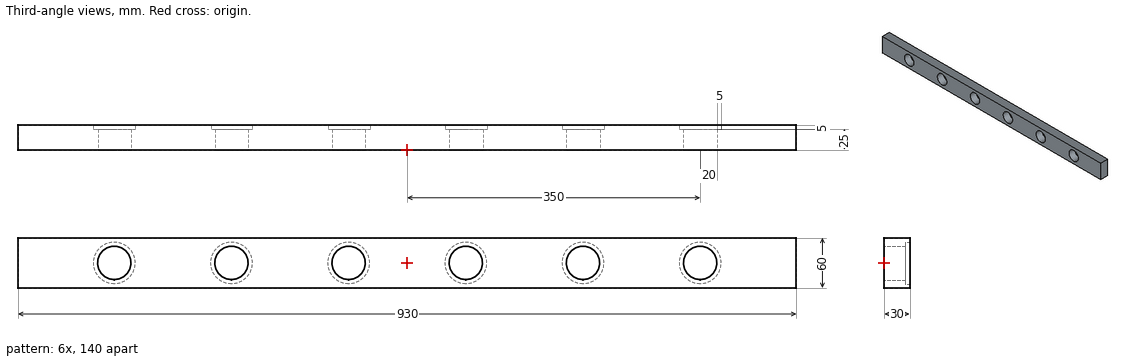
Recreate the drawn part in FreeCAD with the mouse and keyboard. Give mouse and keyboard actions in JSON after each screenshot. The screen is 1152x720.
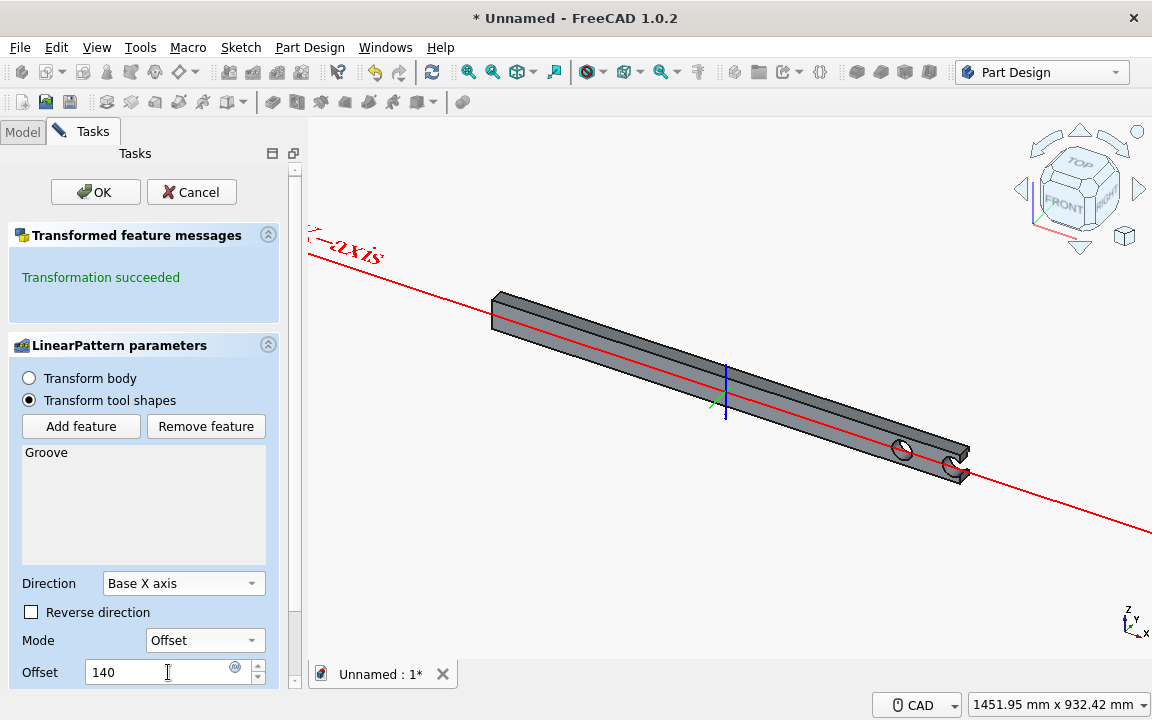
{"action": "scroll", "coordinate": [295, 426], "scroll_direction": "down", "scroll_amount": 2}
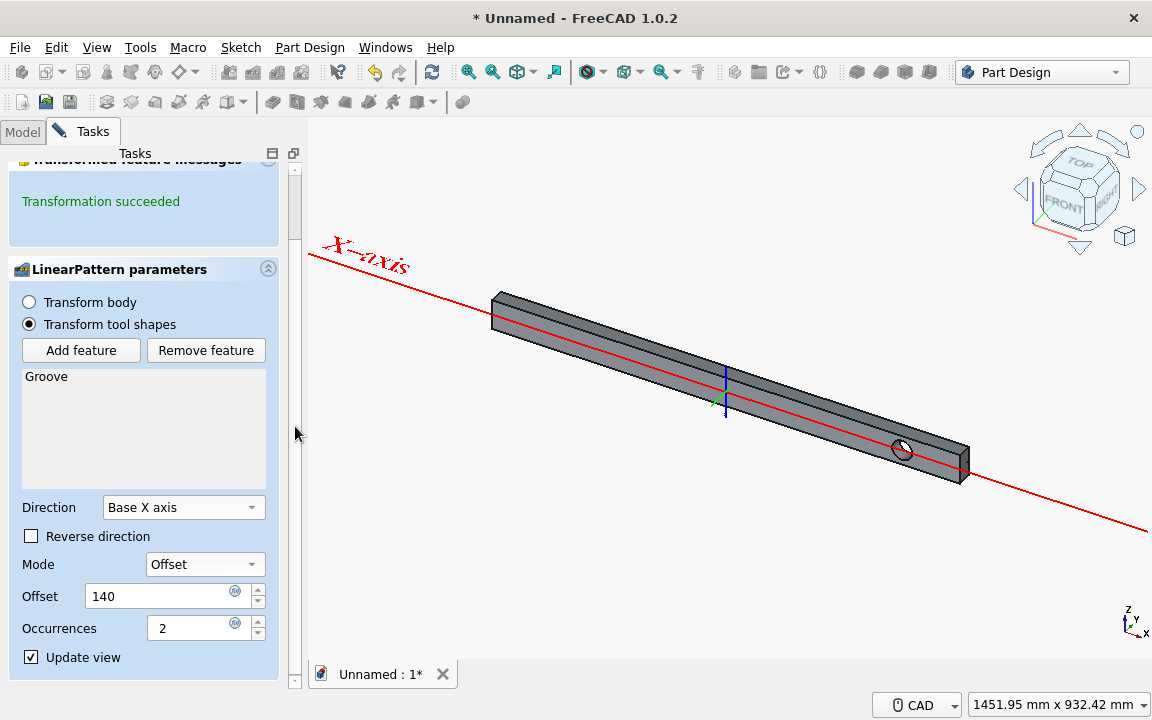
{"action": "triple_click", "coordinate": [198, 628]}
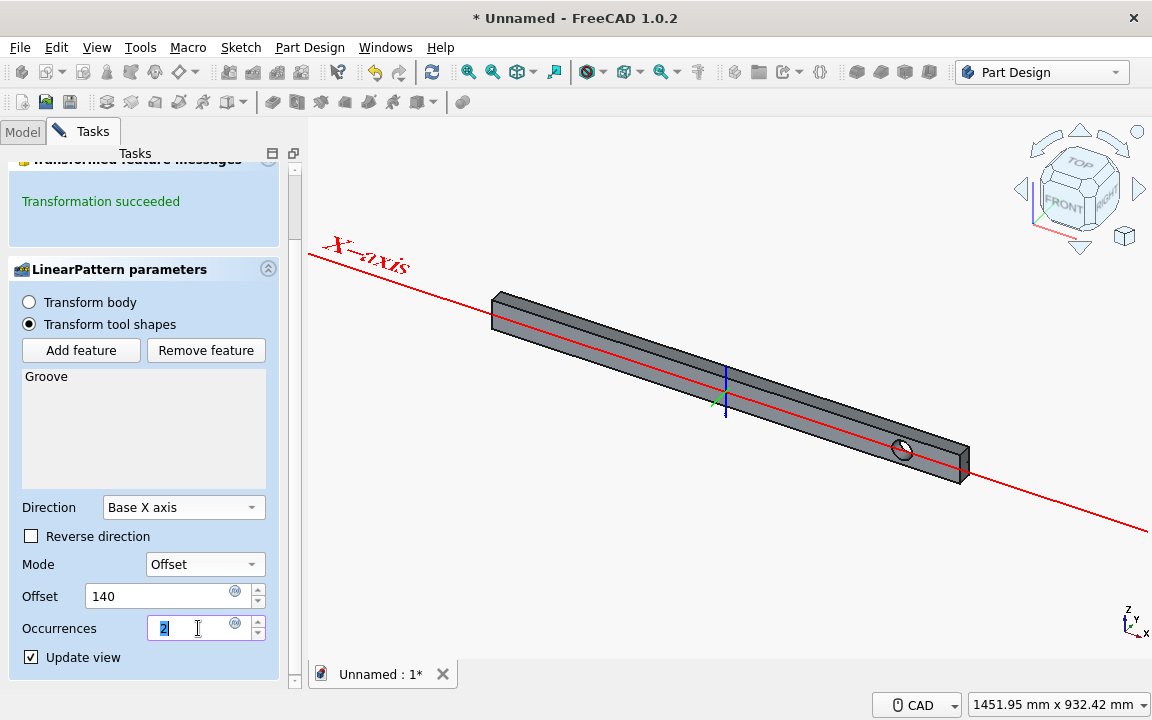
{"action": "type", "text": "6"}
{"action": "key", "text": "Tab"}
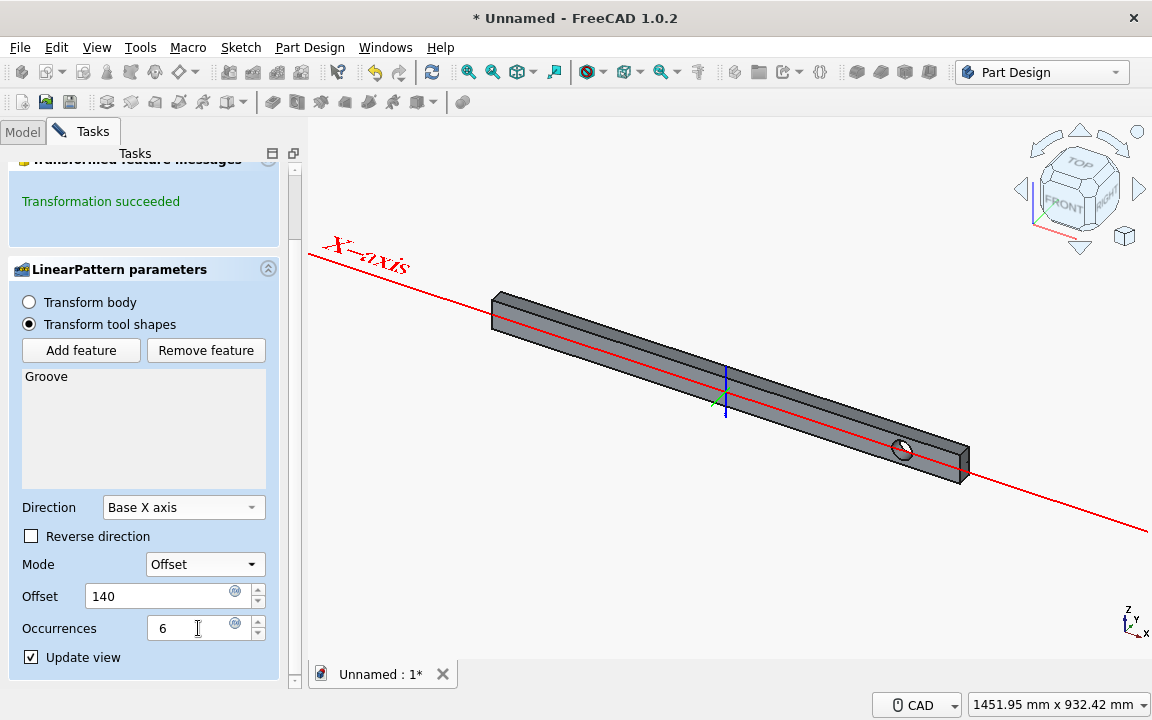
{"action": "left_click", "coordinate": [30, 536]}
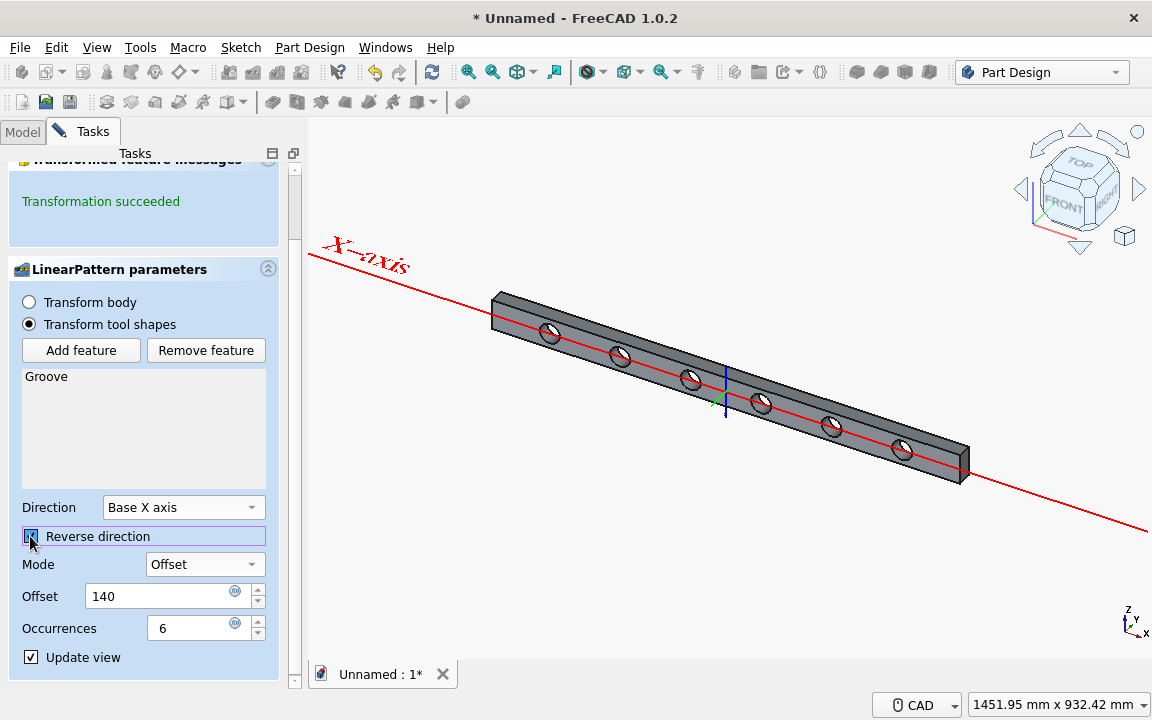
{"action": "scroll", "coordinate": [295, 426], "scroll_direction": "up", "scroll_amount": 3}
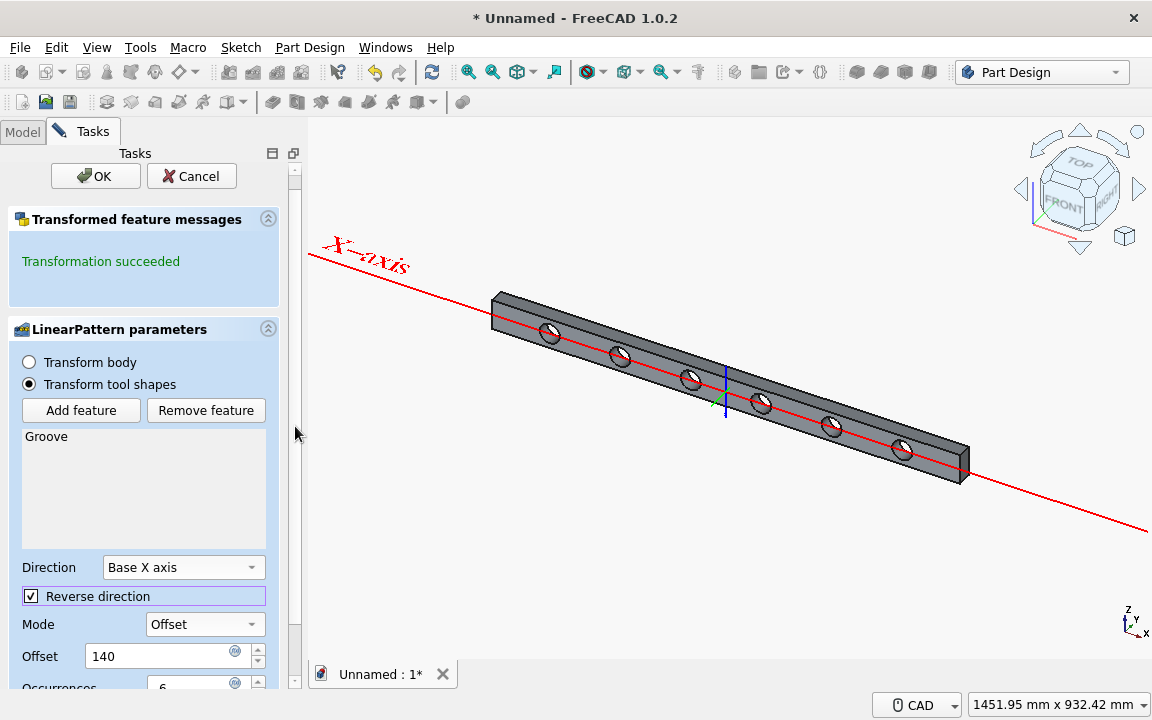
{"action": "left_click", "coordinate": [96, 192]}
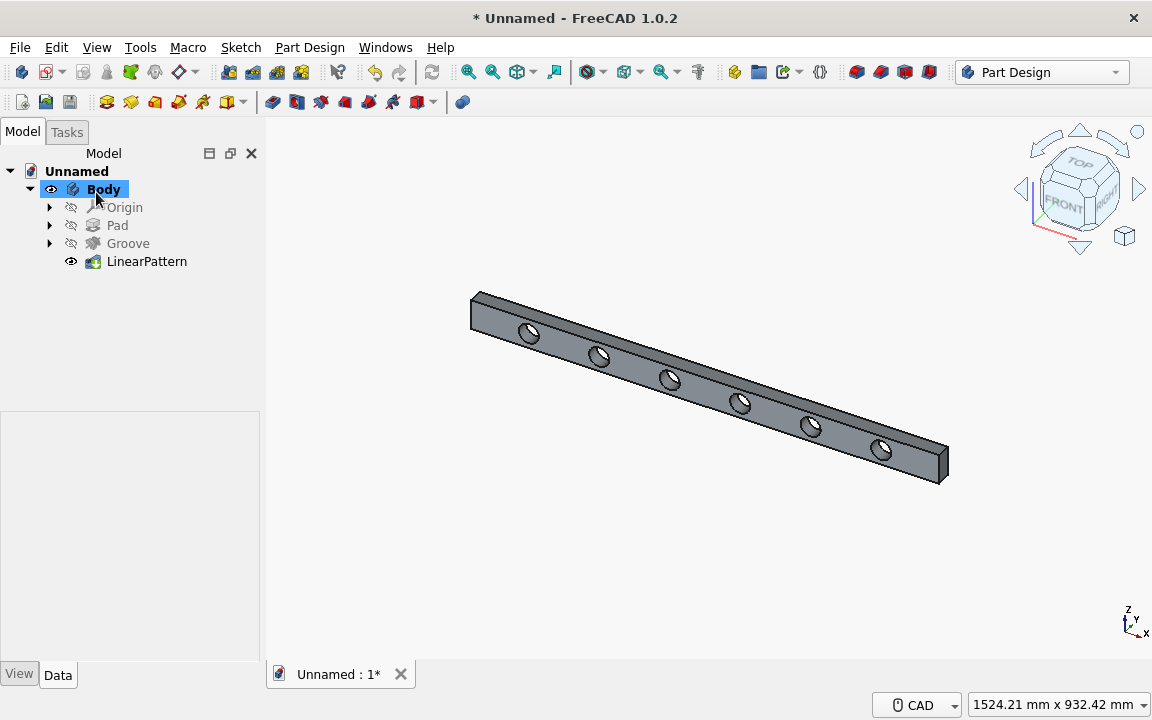
{"action": "key", "text": "0"}